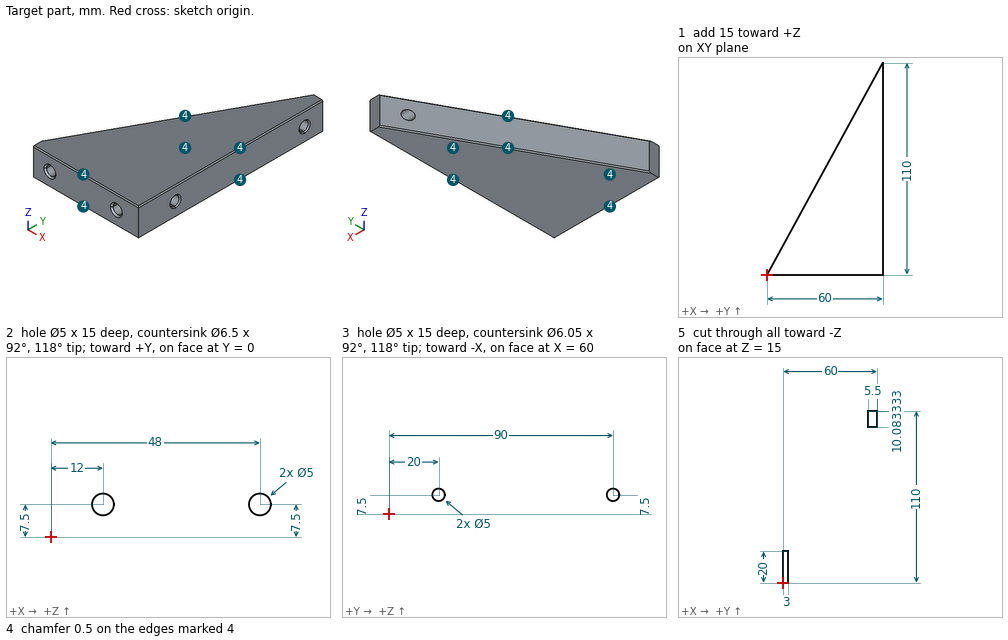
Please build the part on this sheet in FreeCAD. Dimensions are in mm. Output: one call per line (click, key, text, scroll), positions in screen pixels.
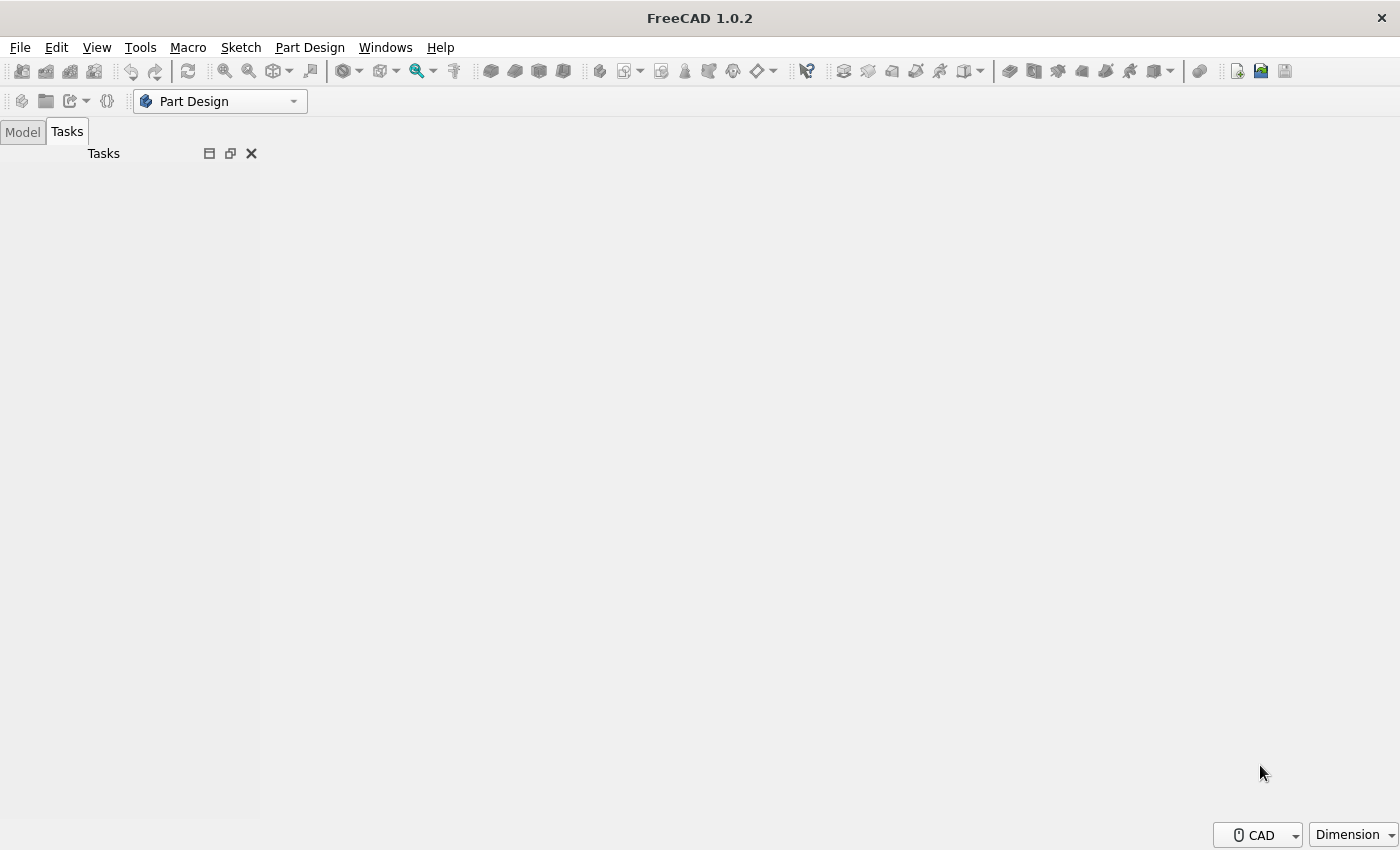
click(1238, 72)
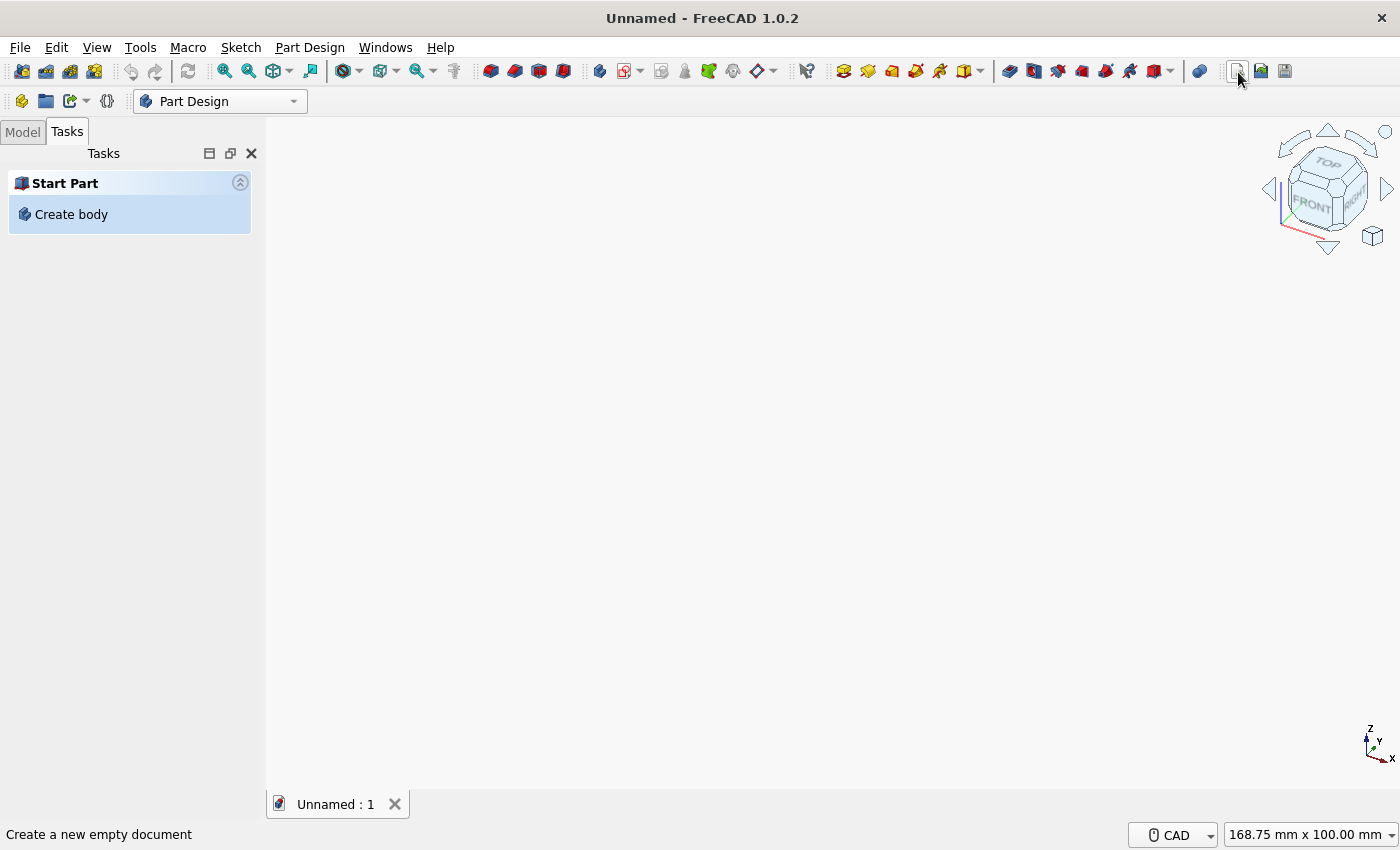
click(624, 72)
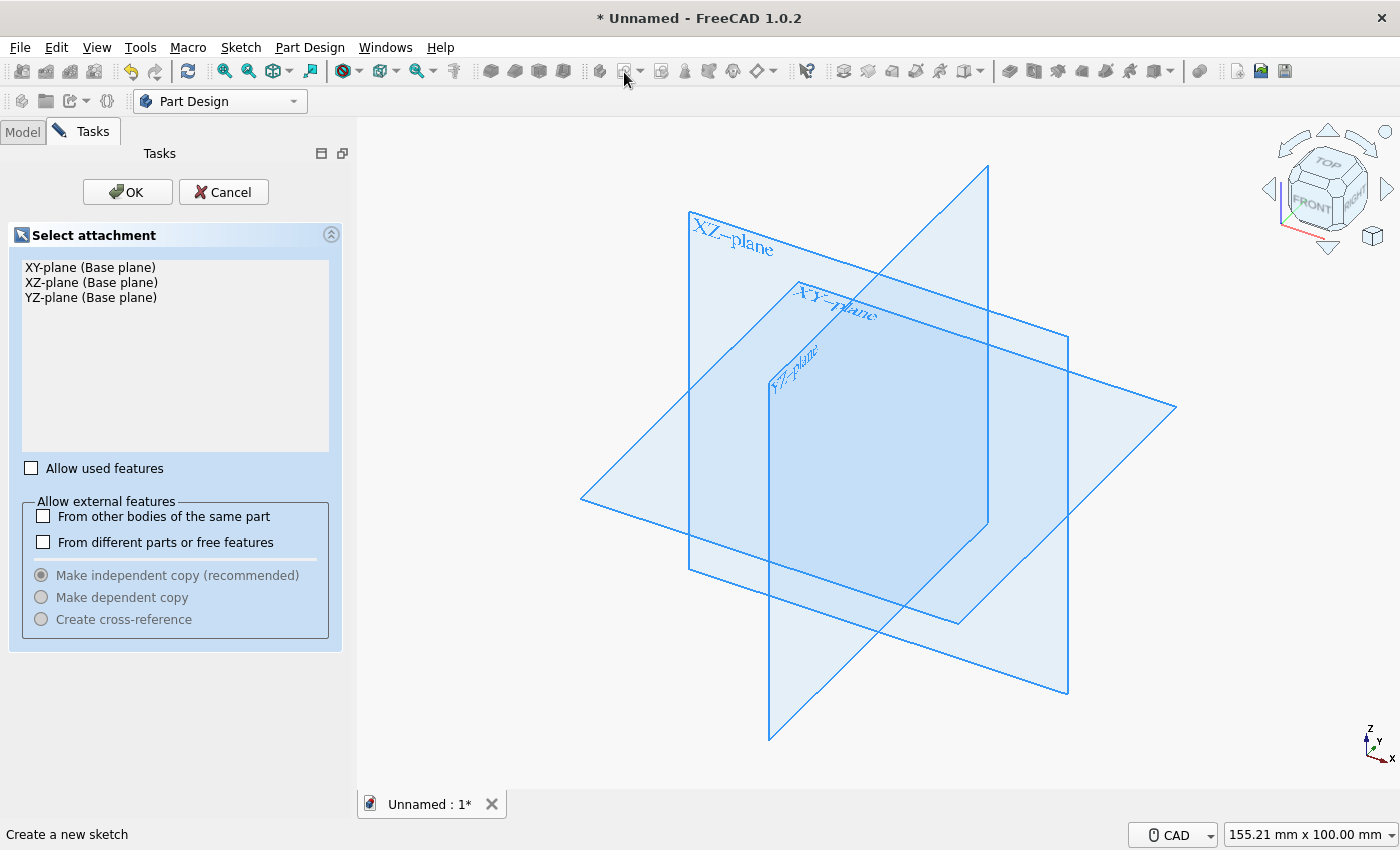
click(82, 268)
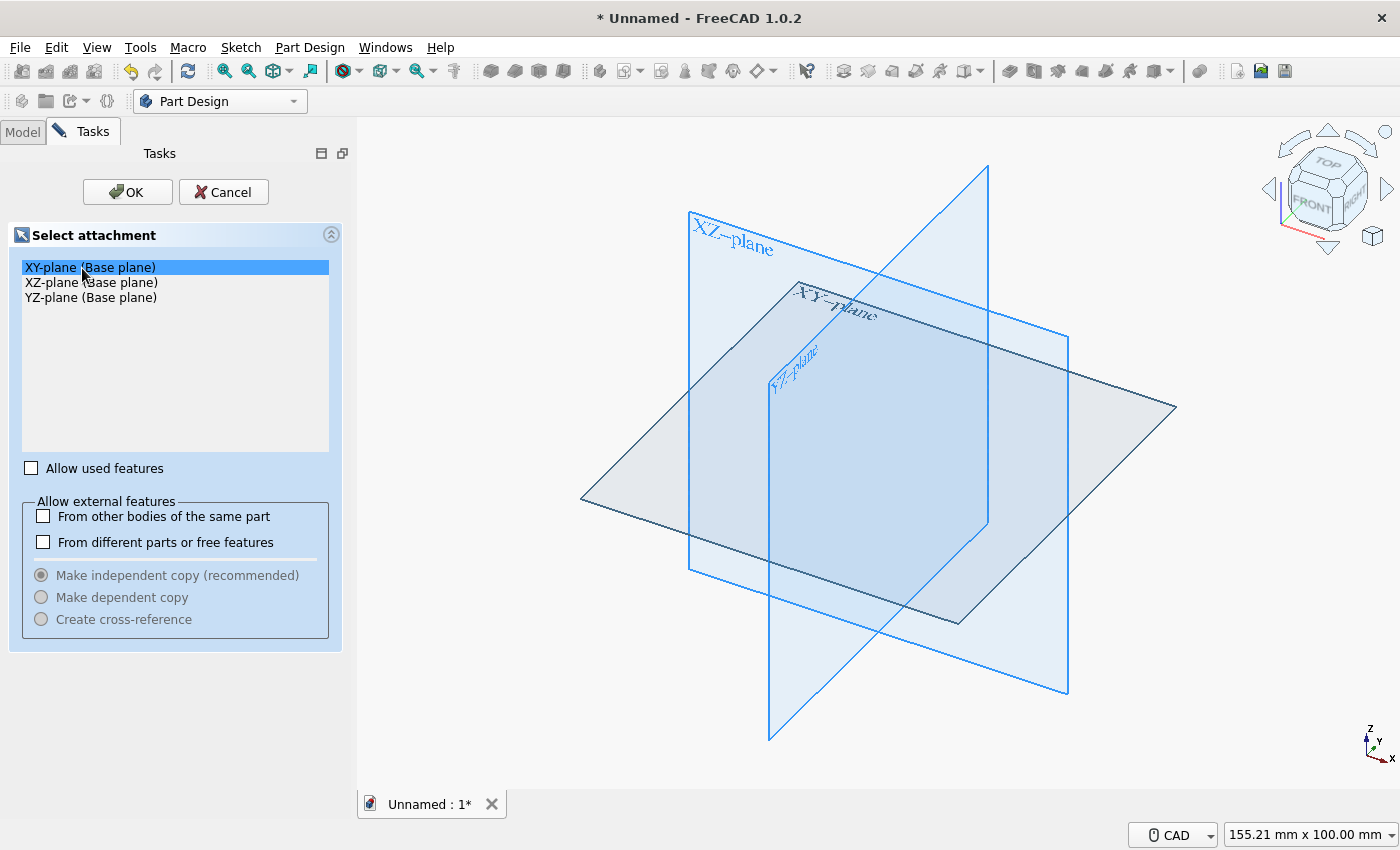
click(128, 192)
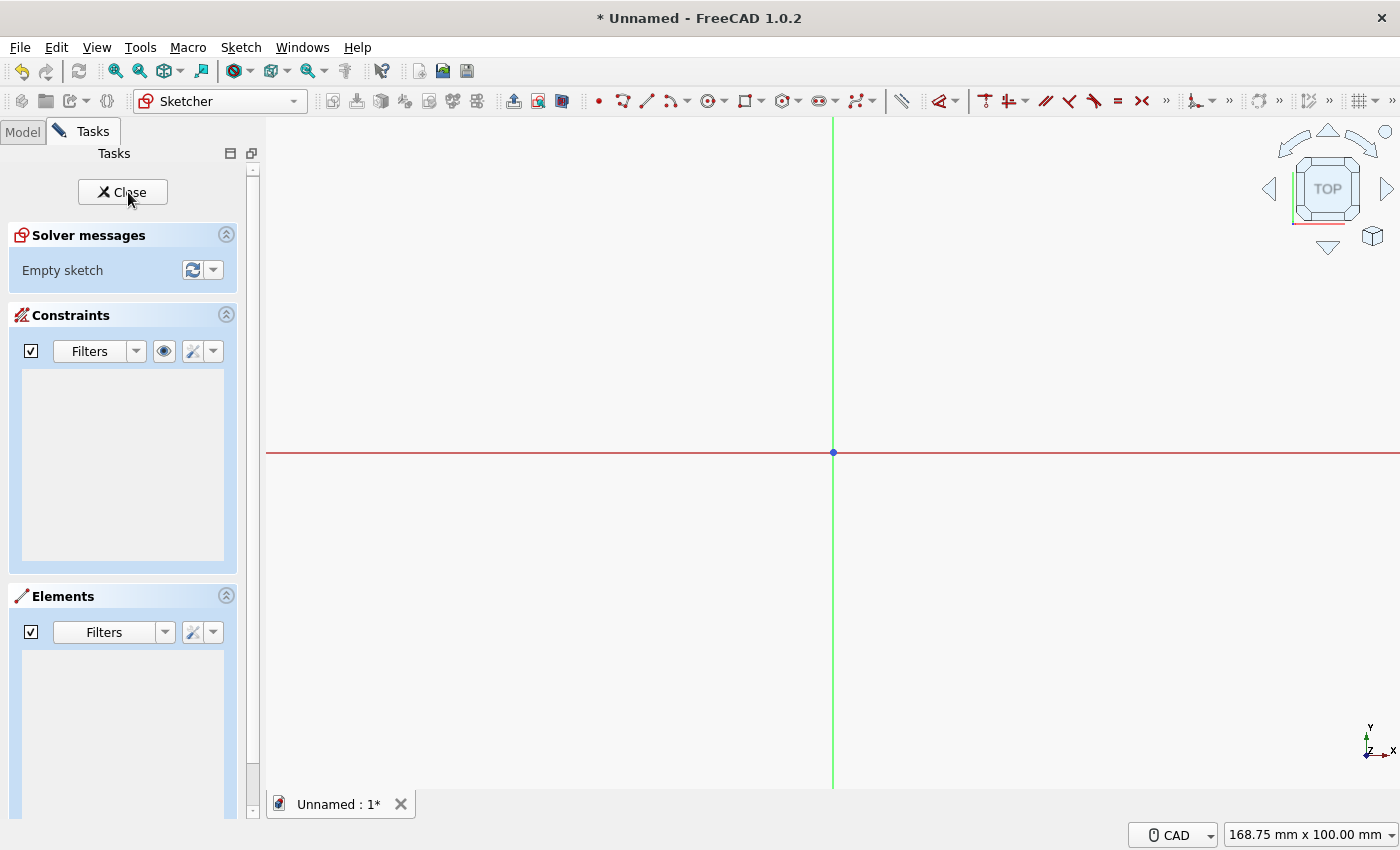
scroll(436, 761, down, 3)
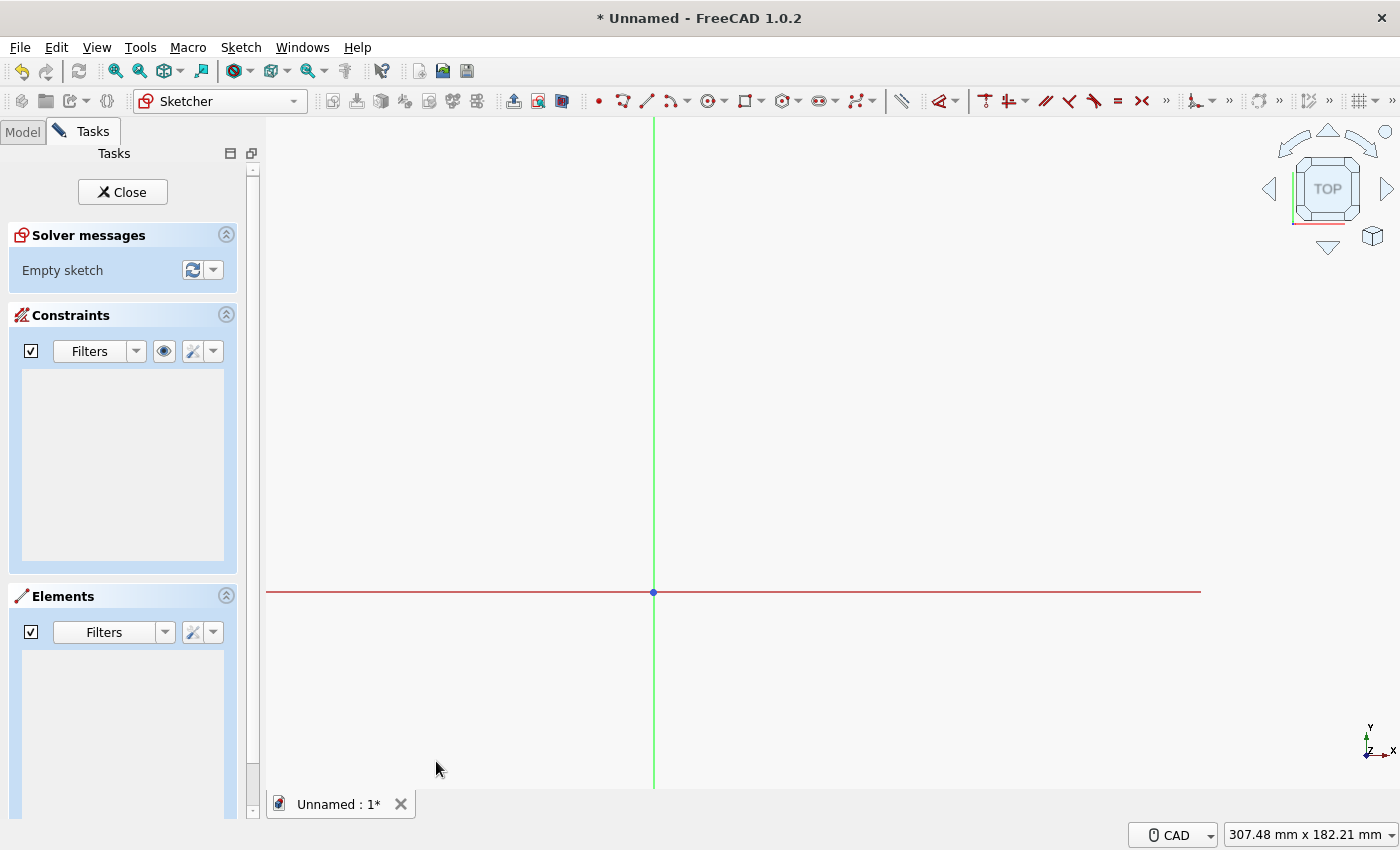
click(624, 102)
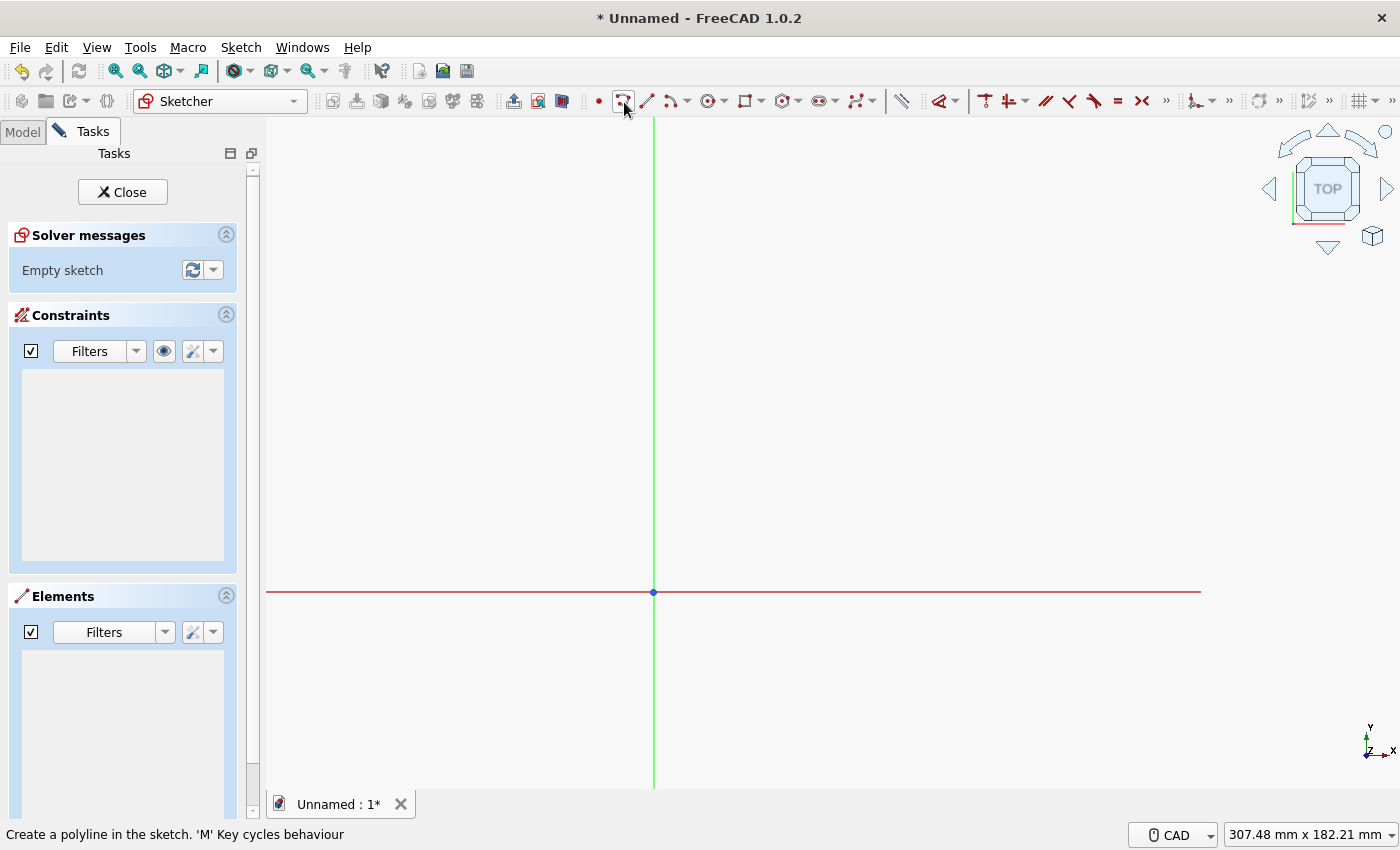
click(654, 592)
click(875, 583)
click(875, 187)
click(654, 592)
key(Escape)
key(Escape)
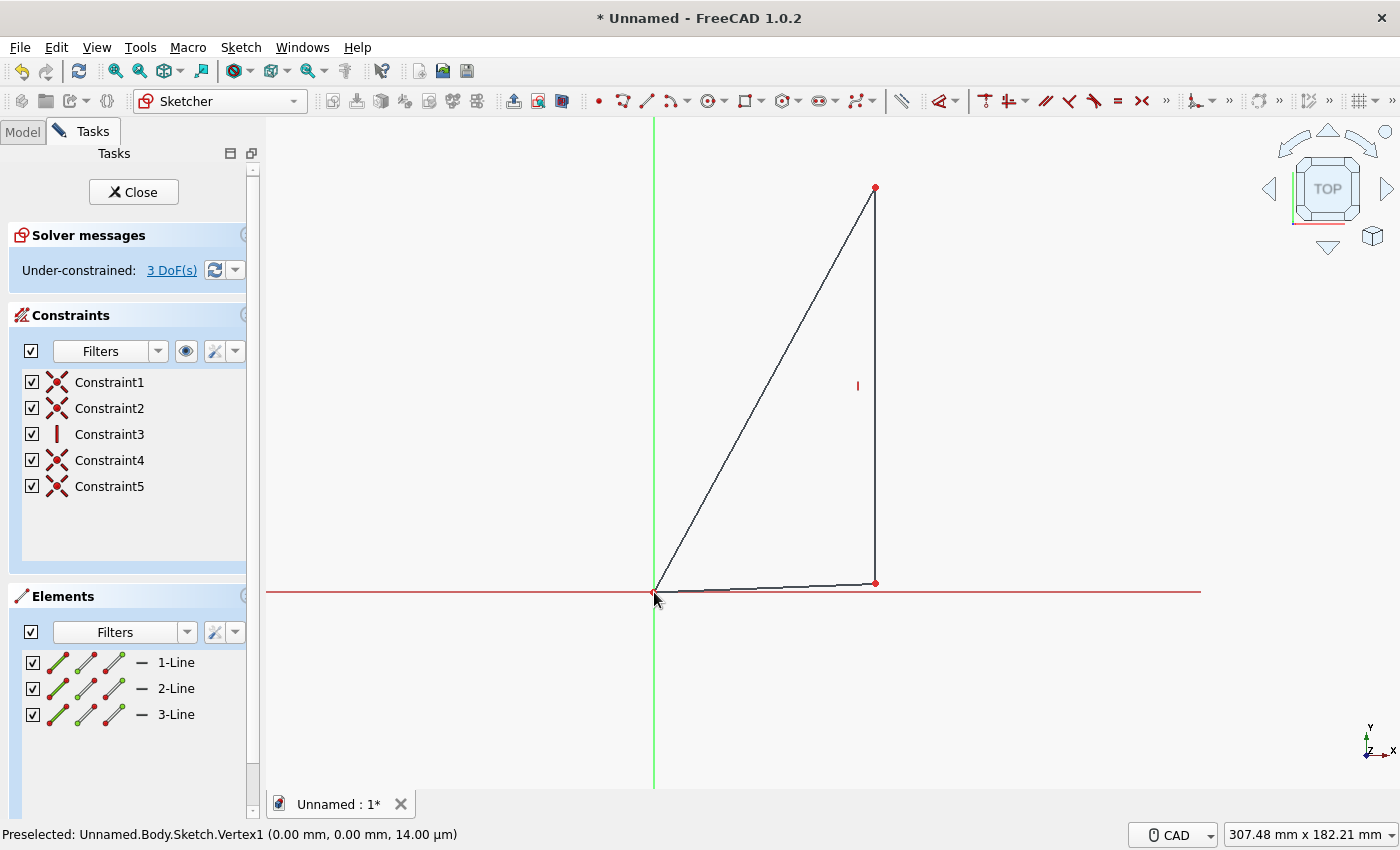
click(720, 590)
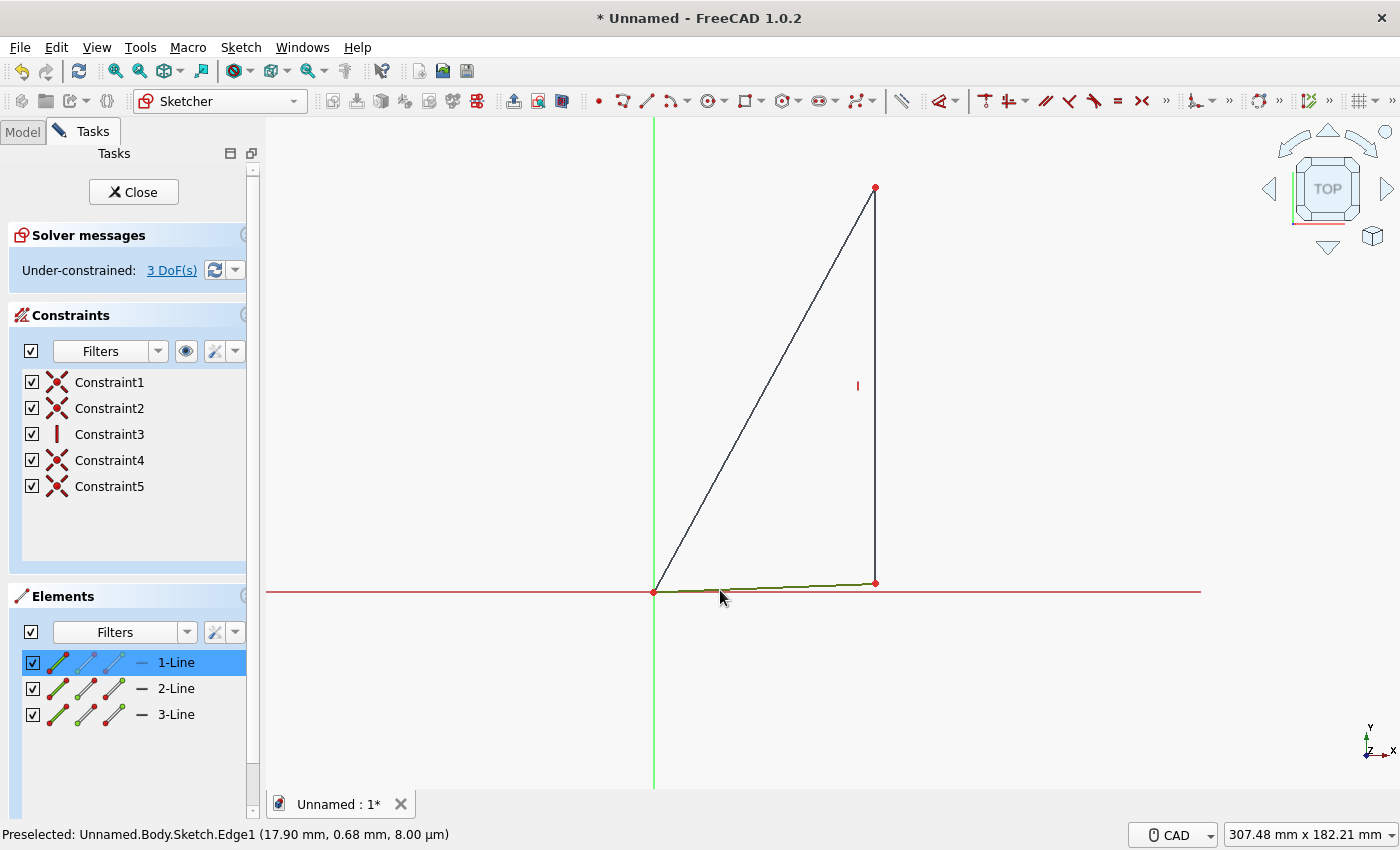
click(1028, 102)